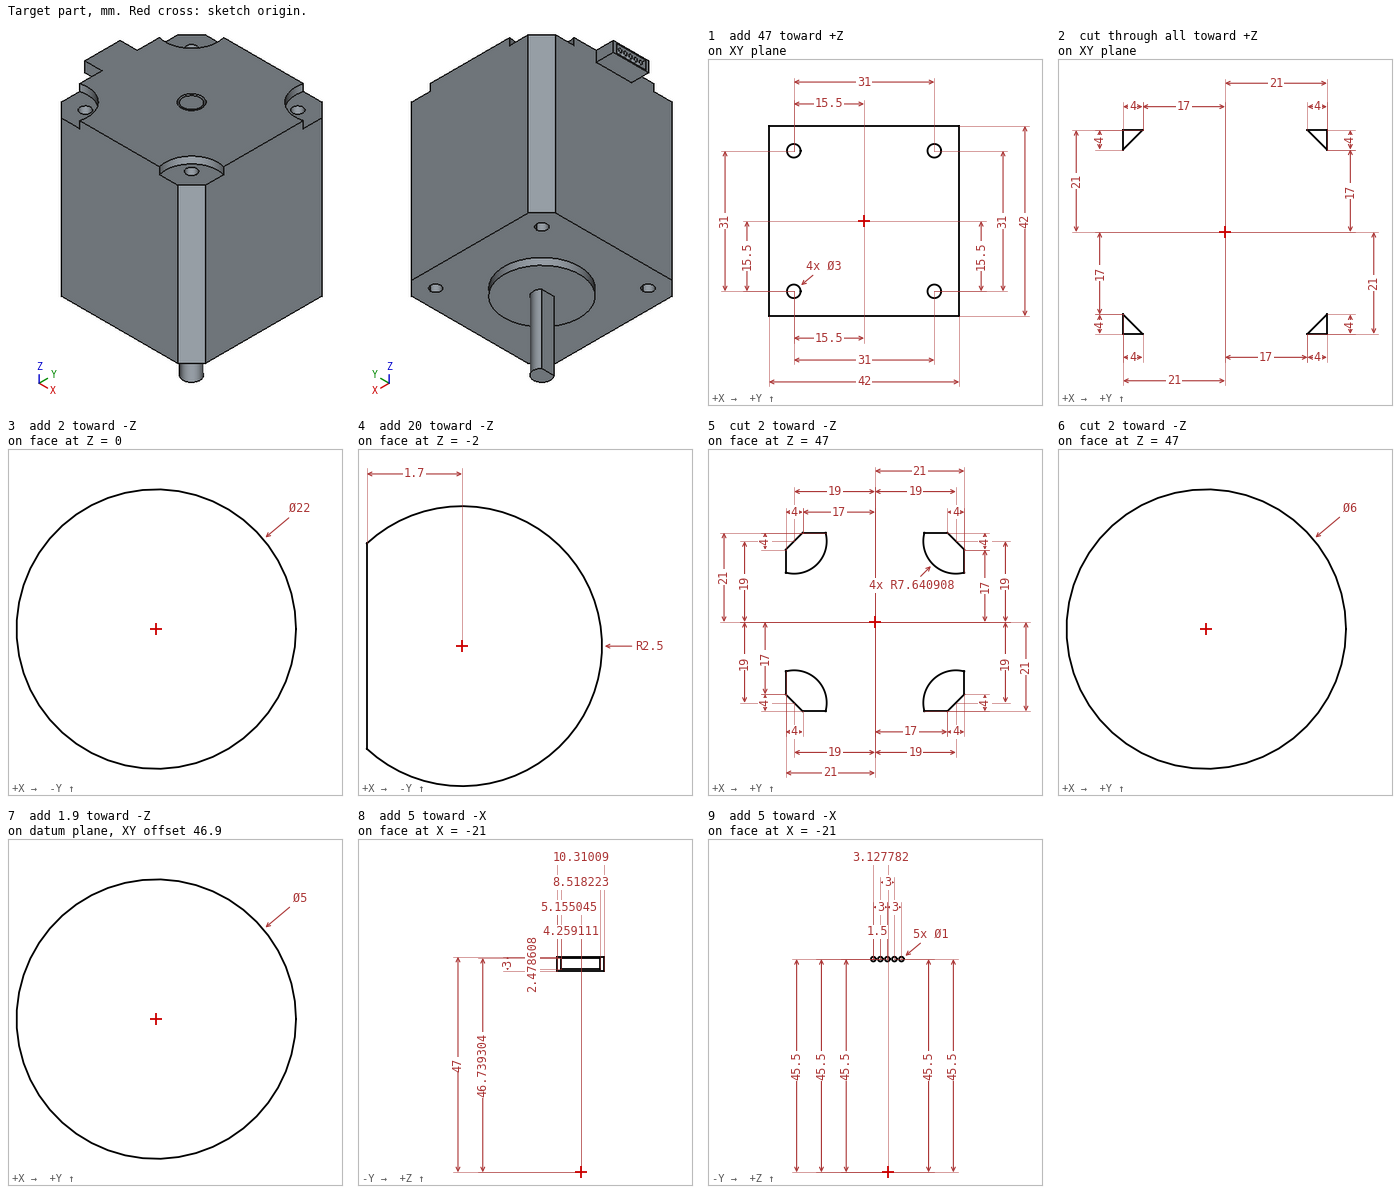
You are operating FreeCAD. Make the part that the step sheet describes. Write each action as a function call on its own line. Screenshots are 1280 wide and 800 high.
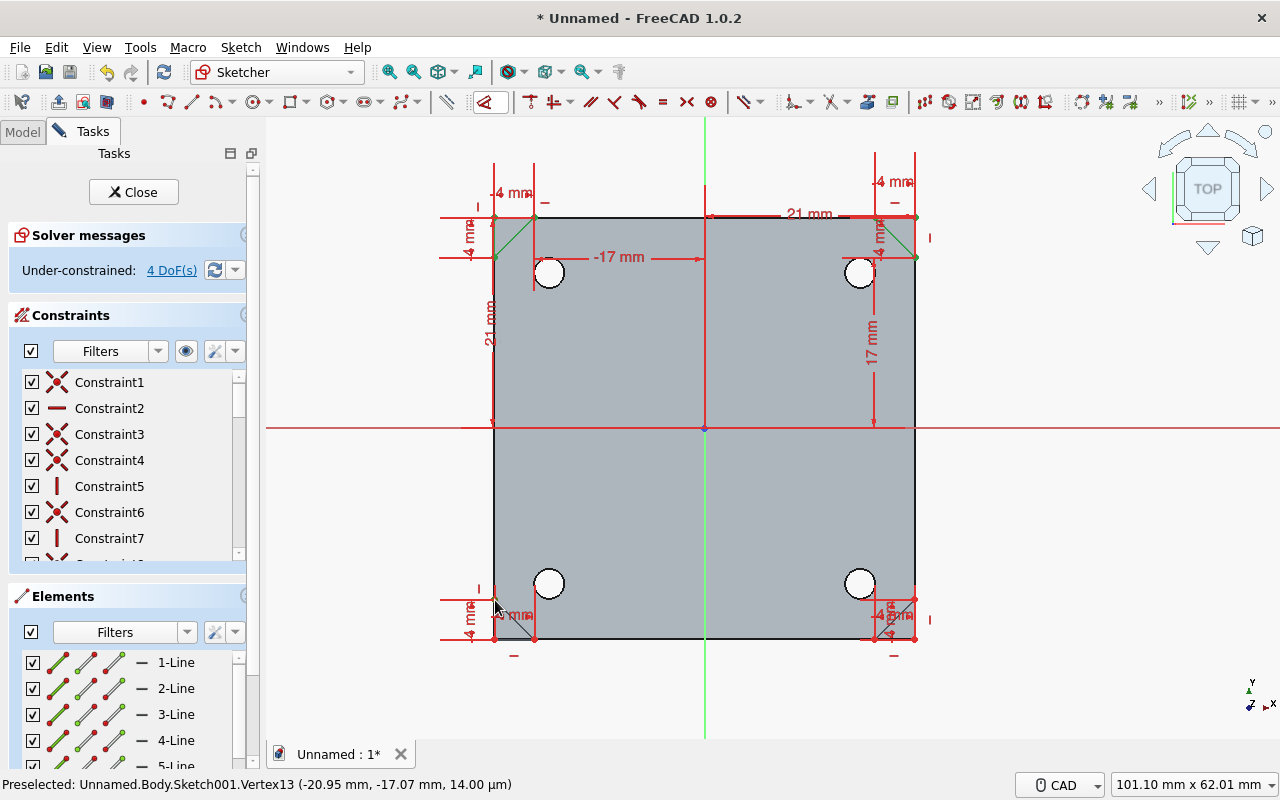
click(502, 102)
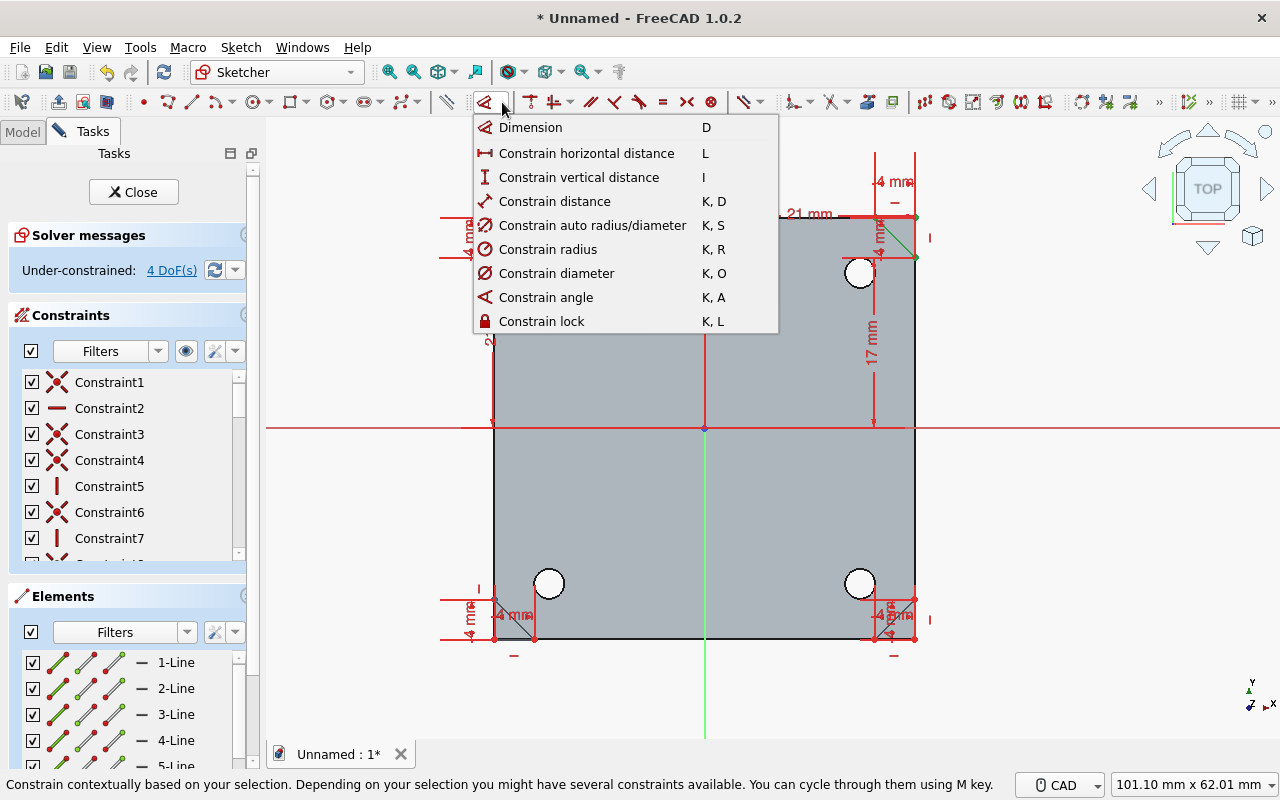
click(626, 153)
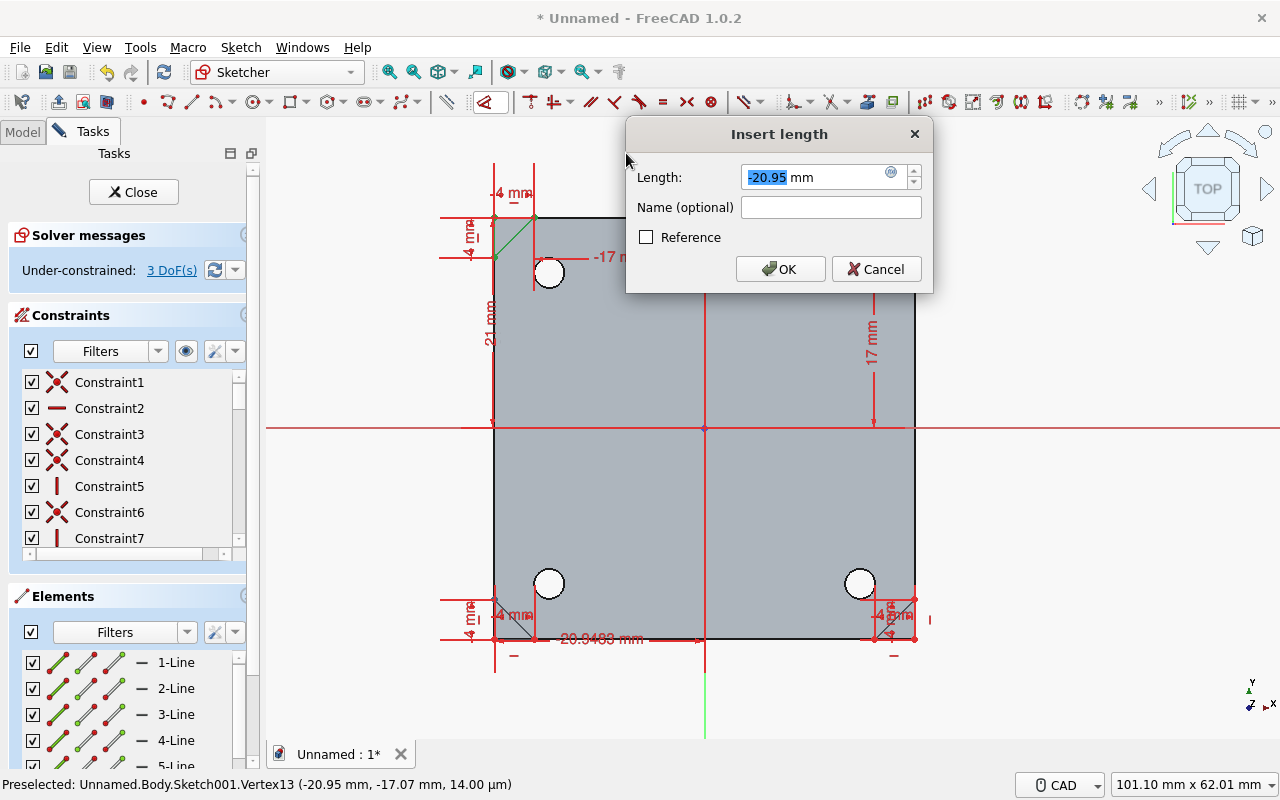
text(-21)
key(Return)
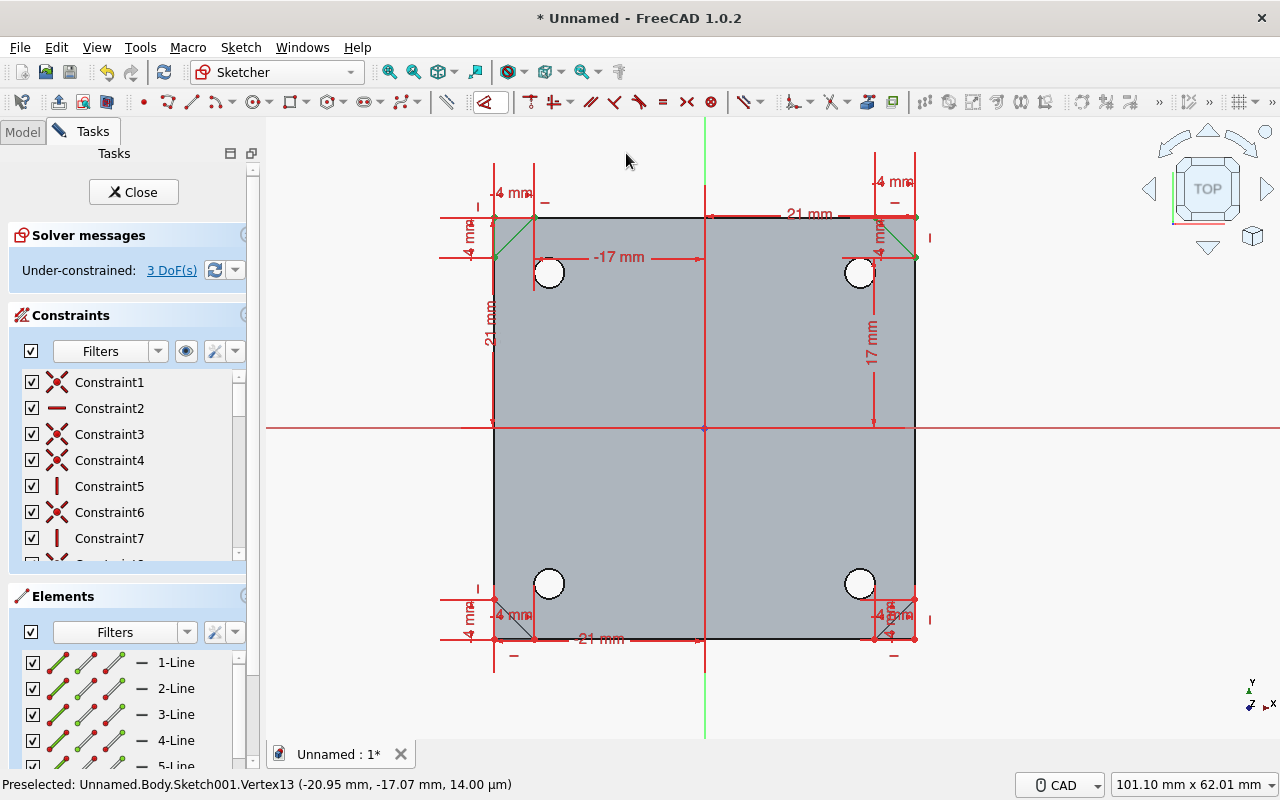
click(494, 600)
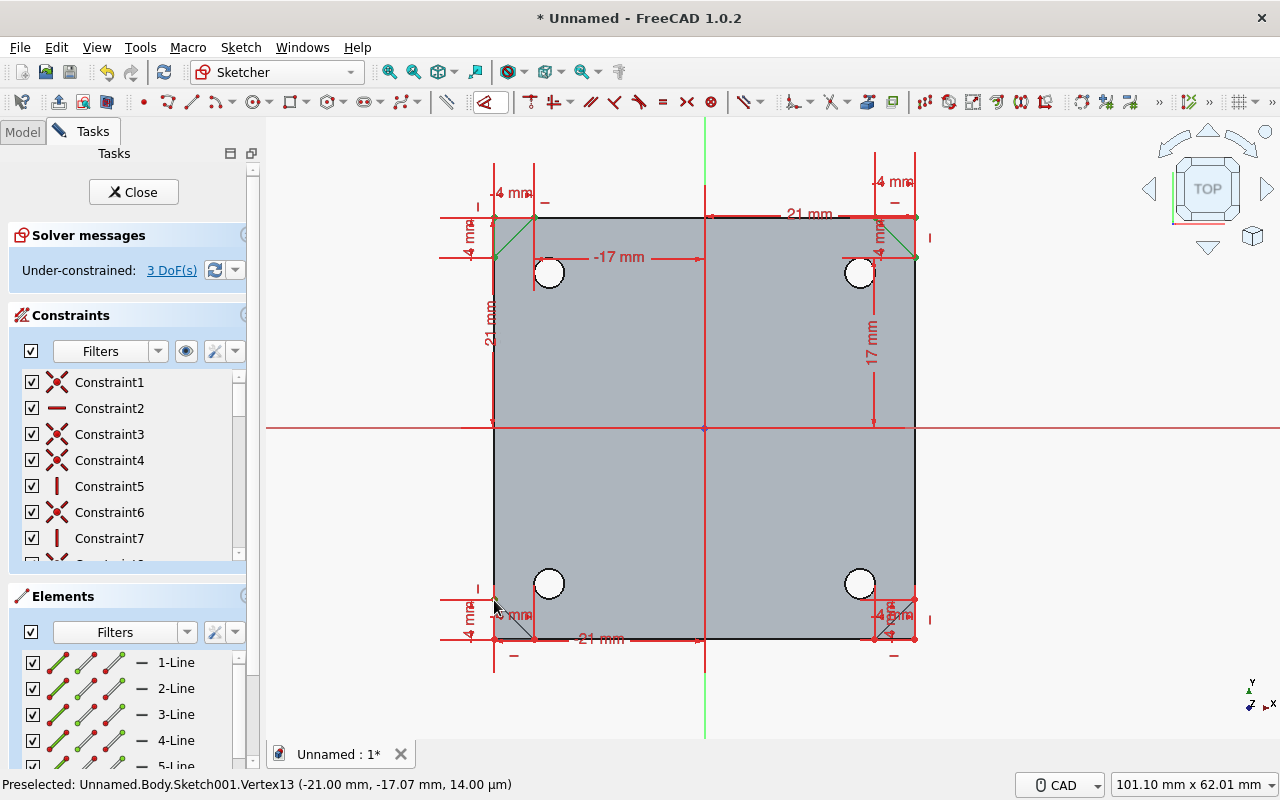
key(i)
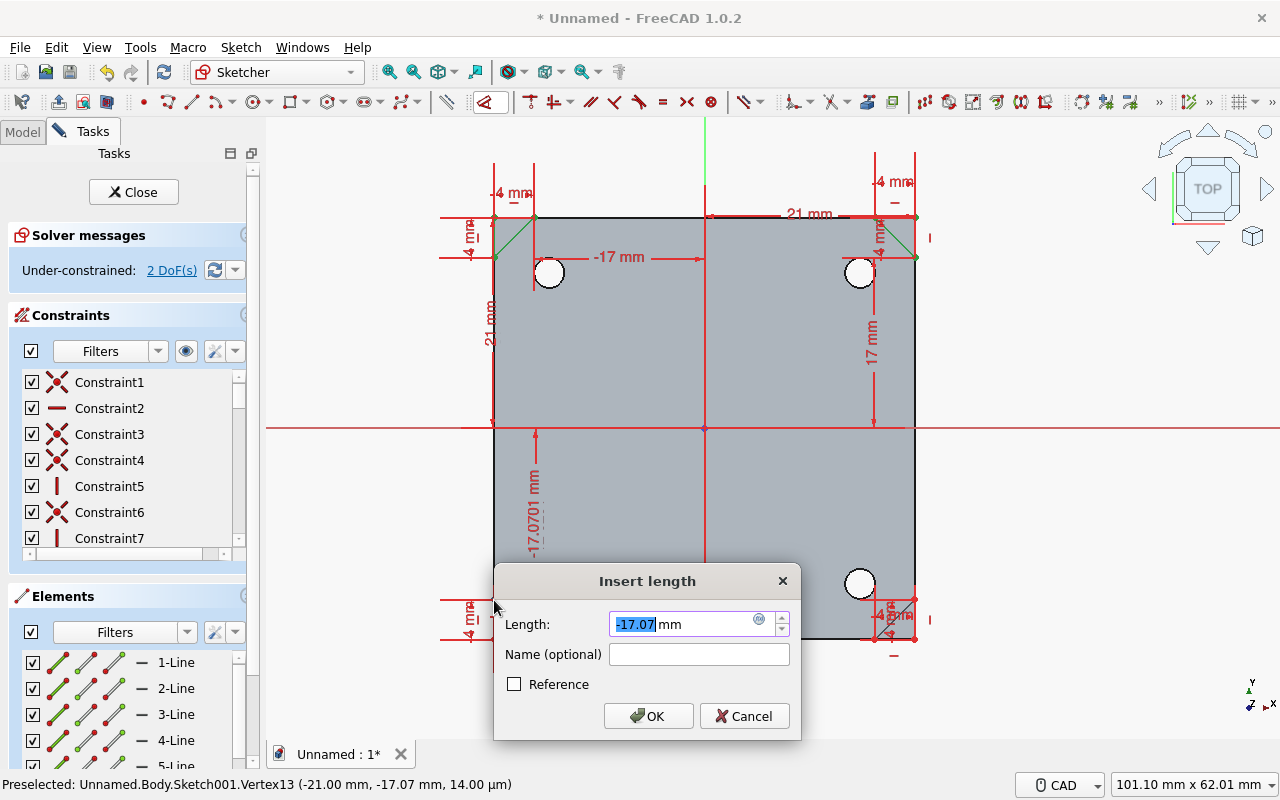
text(-17)
key(Return)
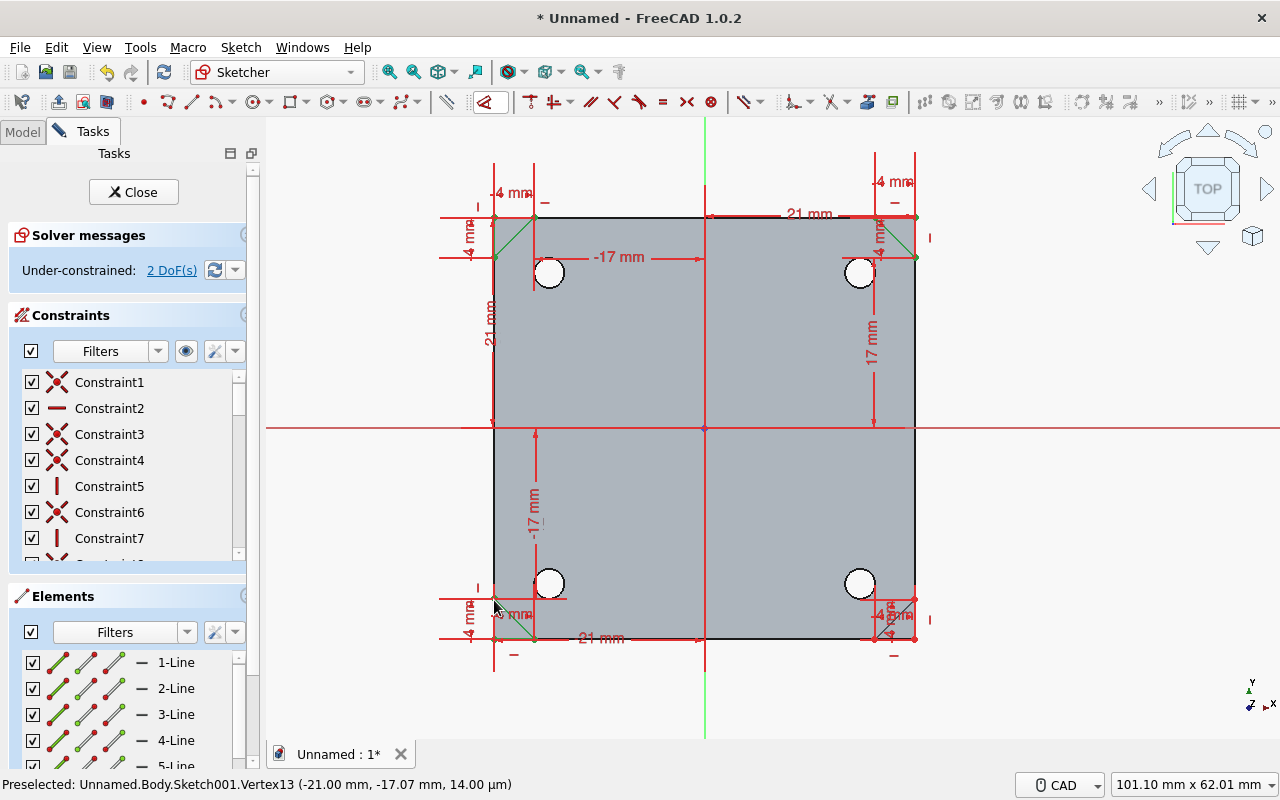
click(875, 640)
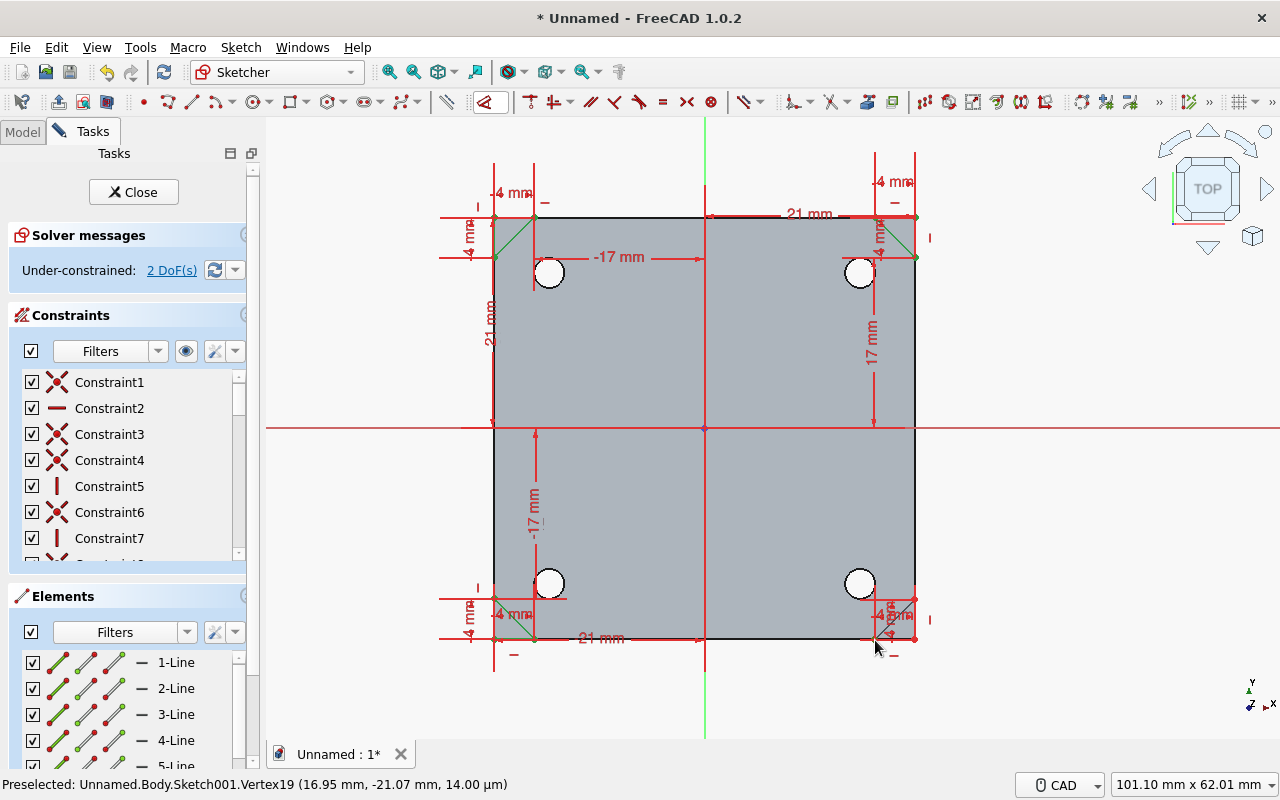
click(502, 102)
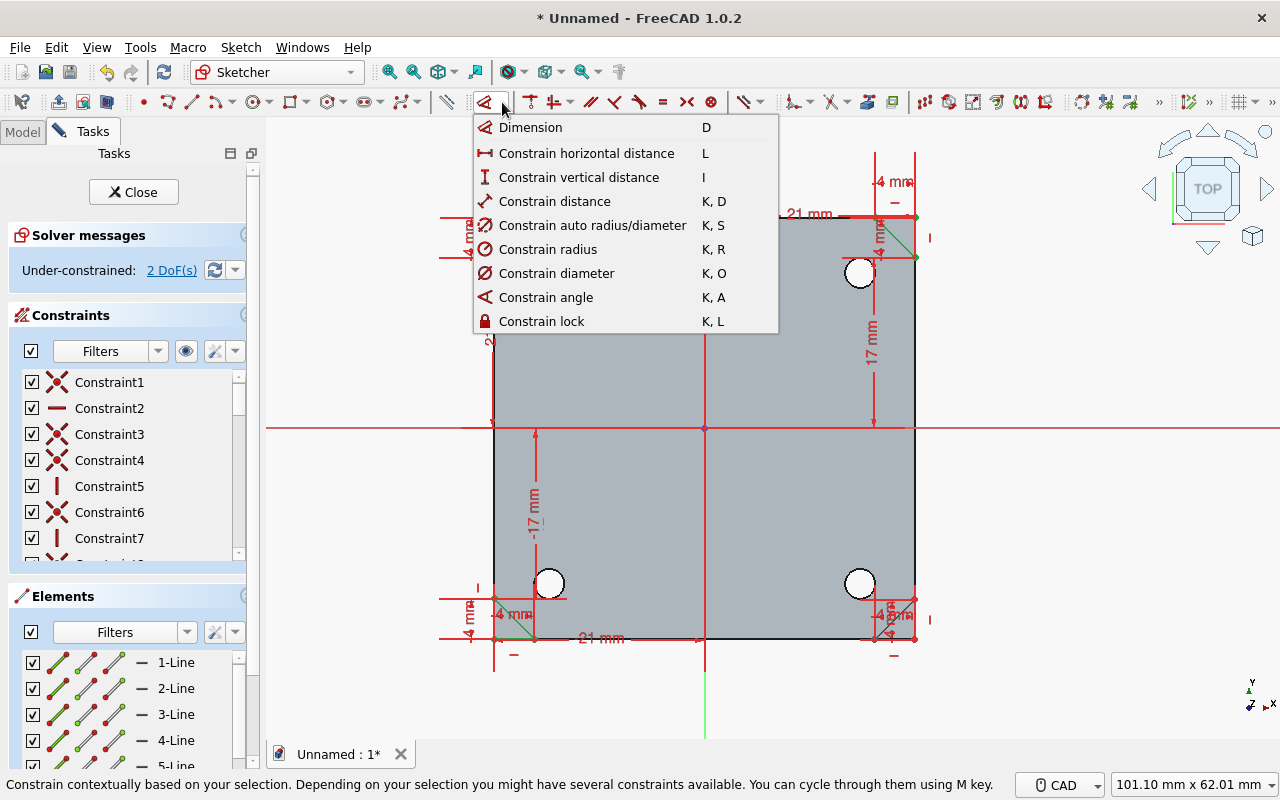
click(626, 153)